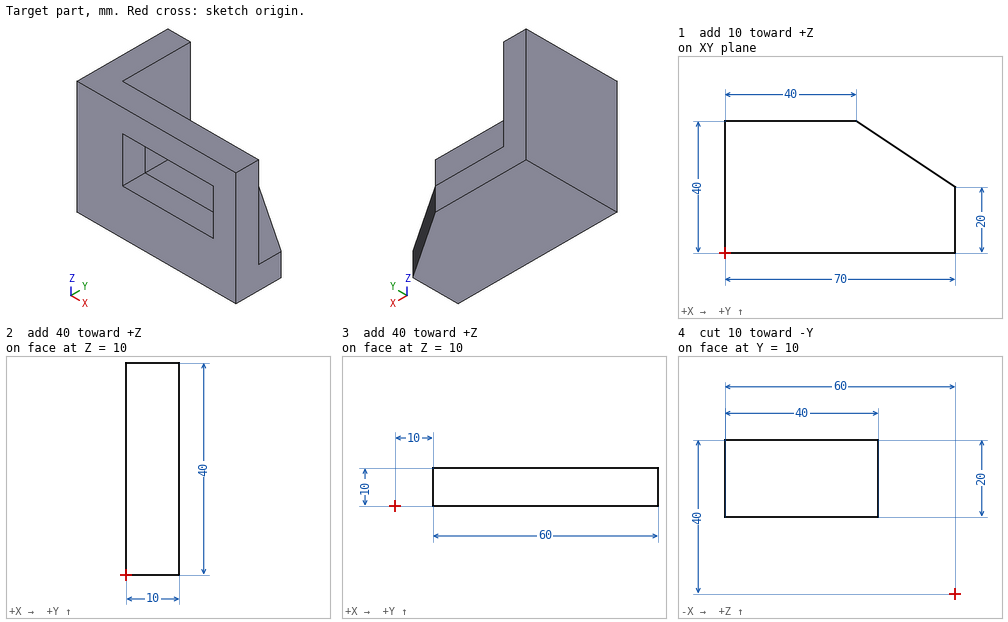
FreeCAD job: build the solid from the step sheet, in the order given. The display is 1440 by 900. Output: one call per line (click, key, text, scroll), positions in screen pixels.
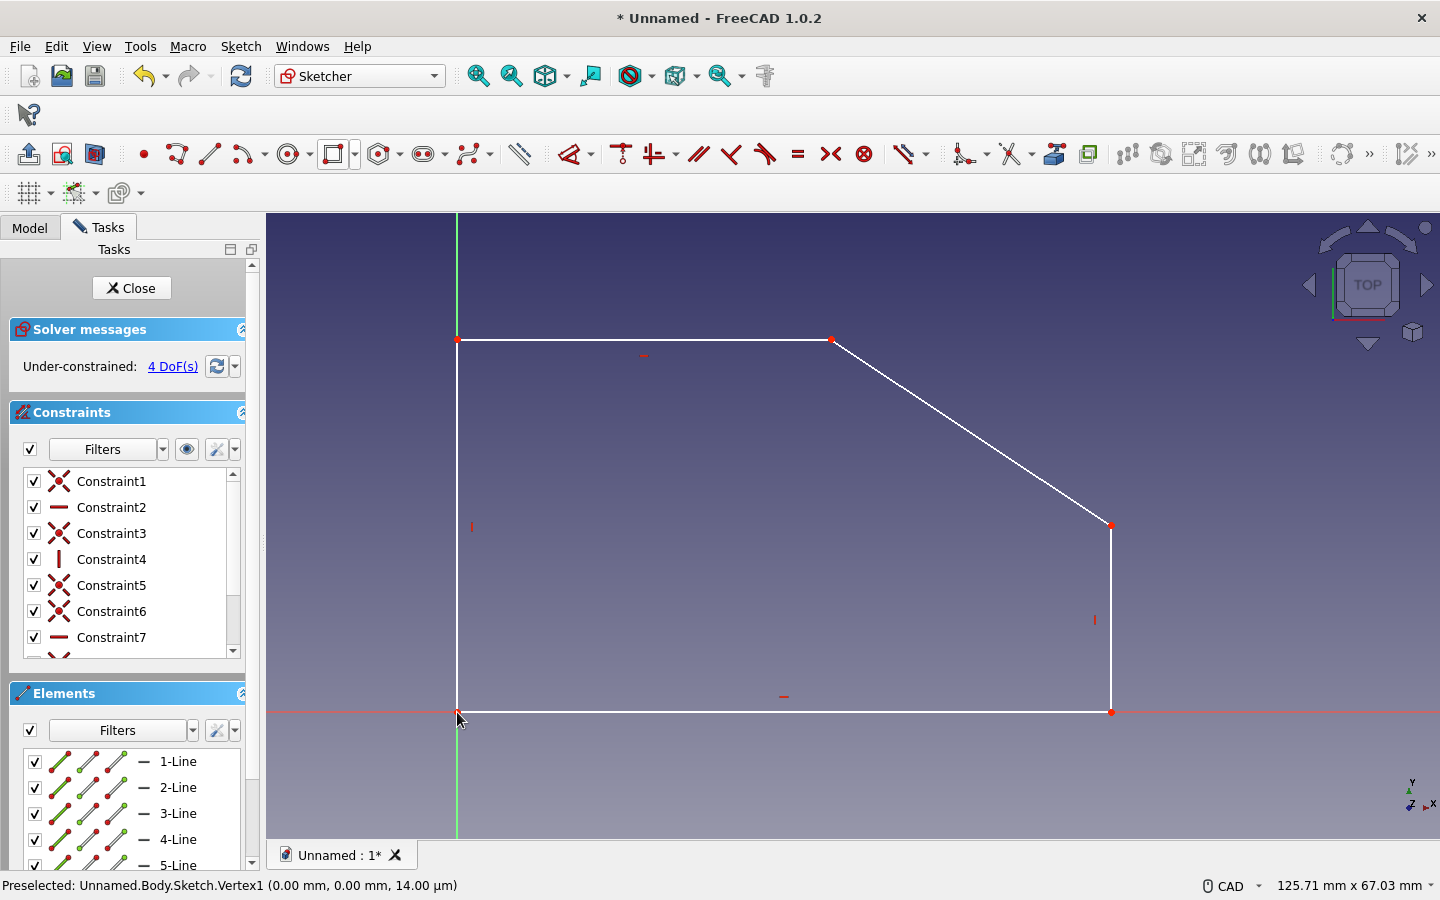
click(568, 154)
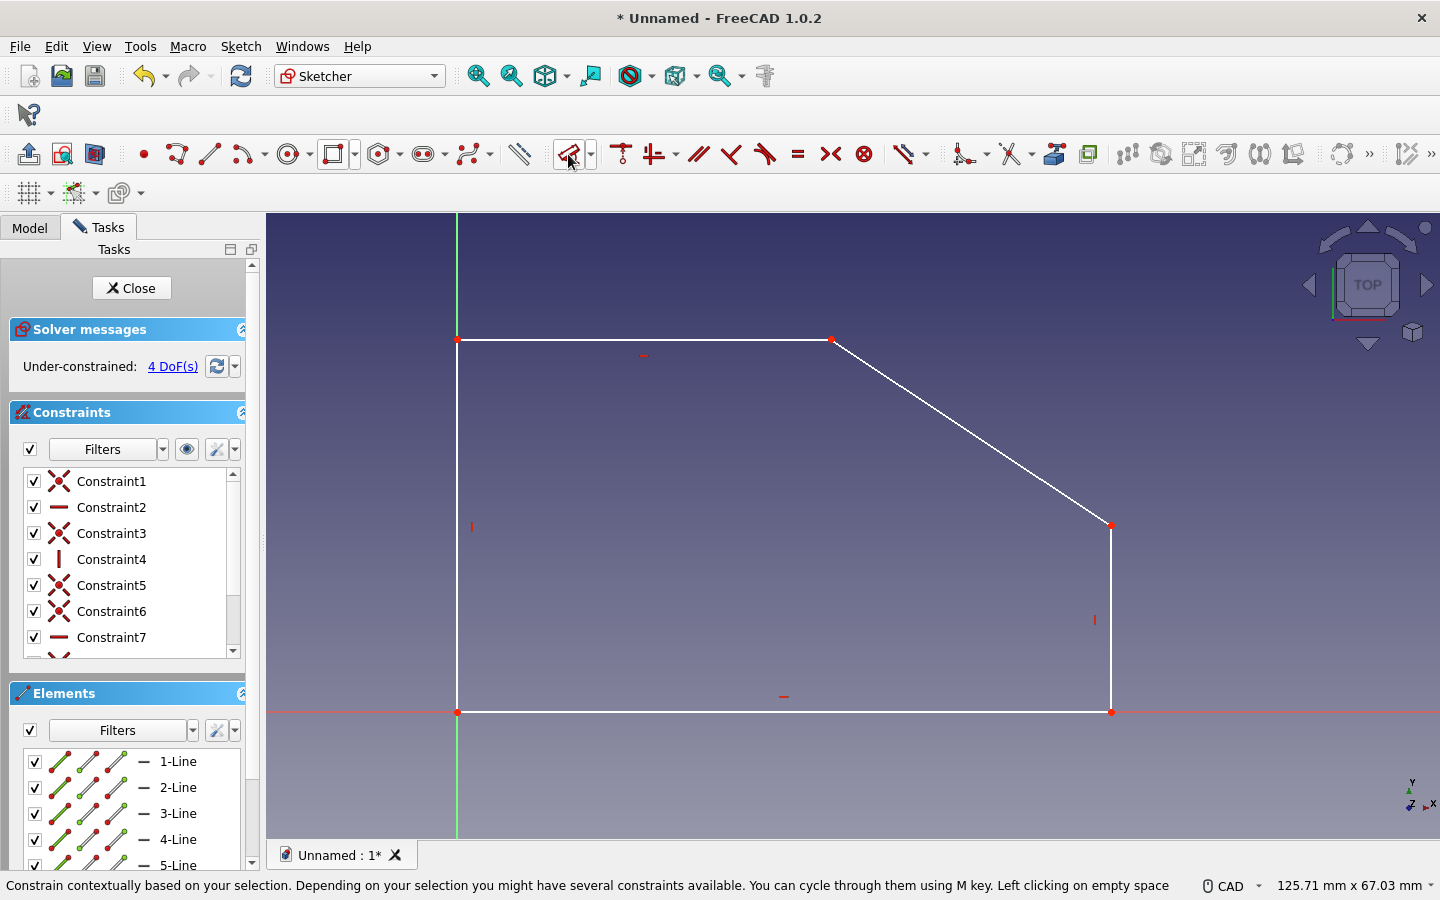
click(653, 712)
click(784, 746)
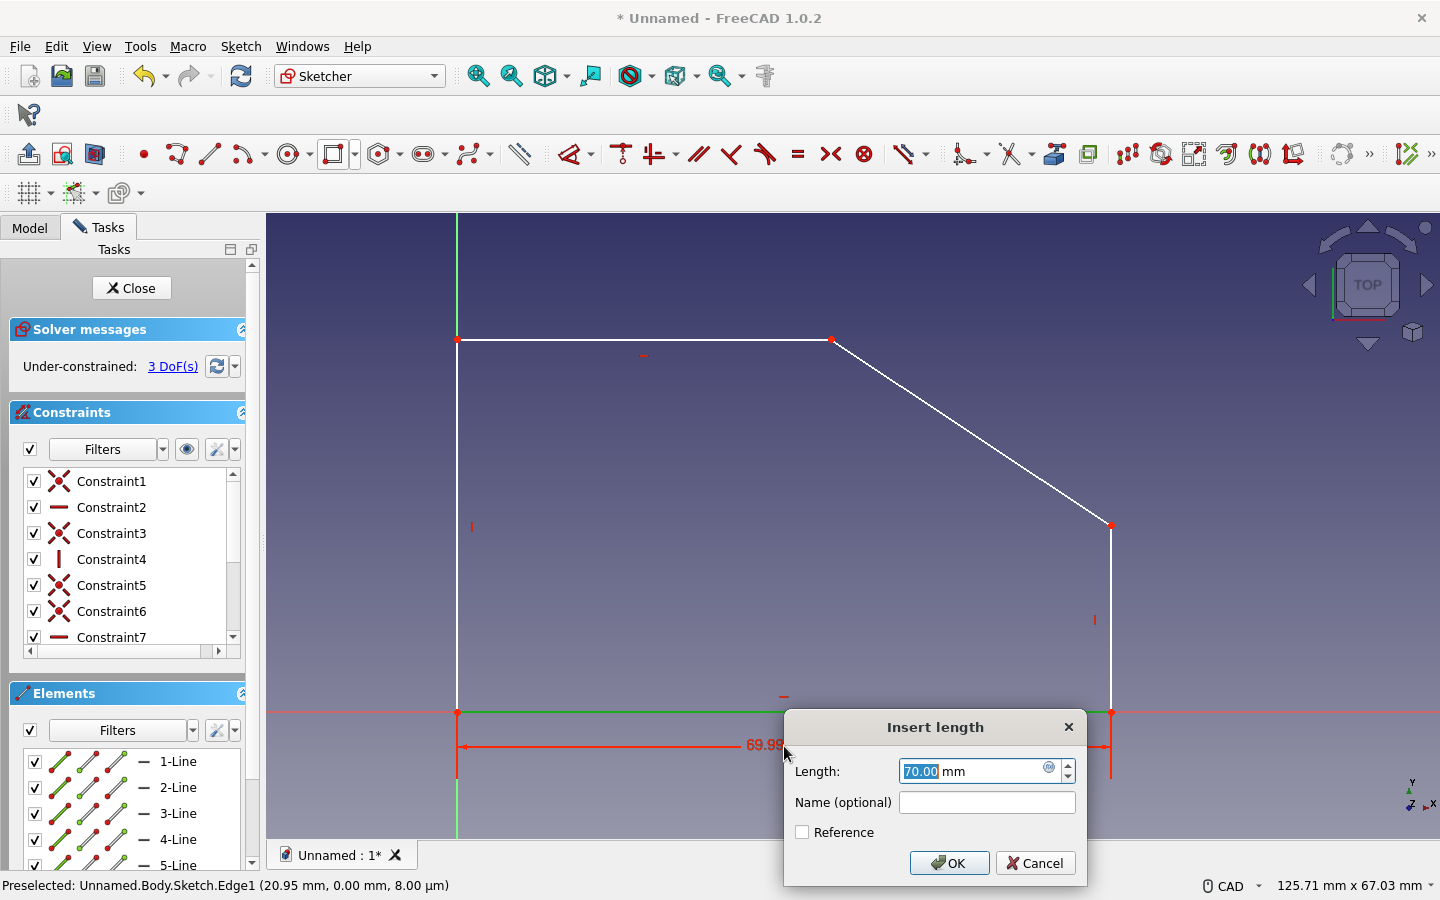
text(70)
key(Return)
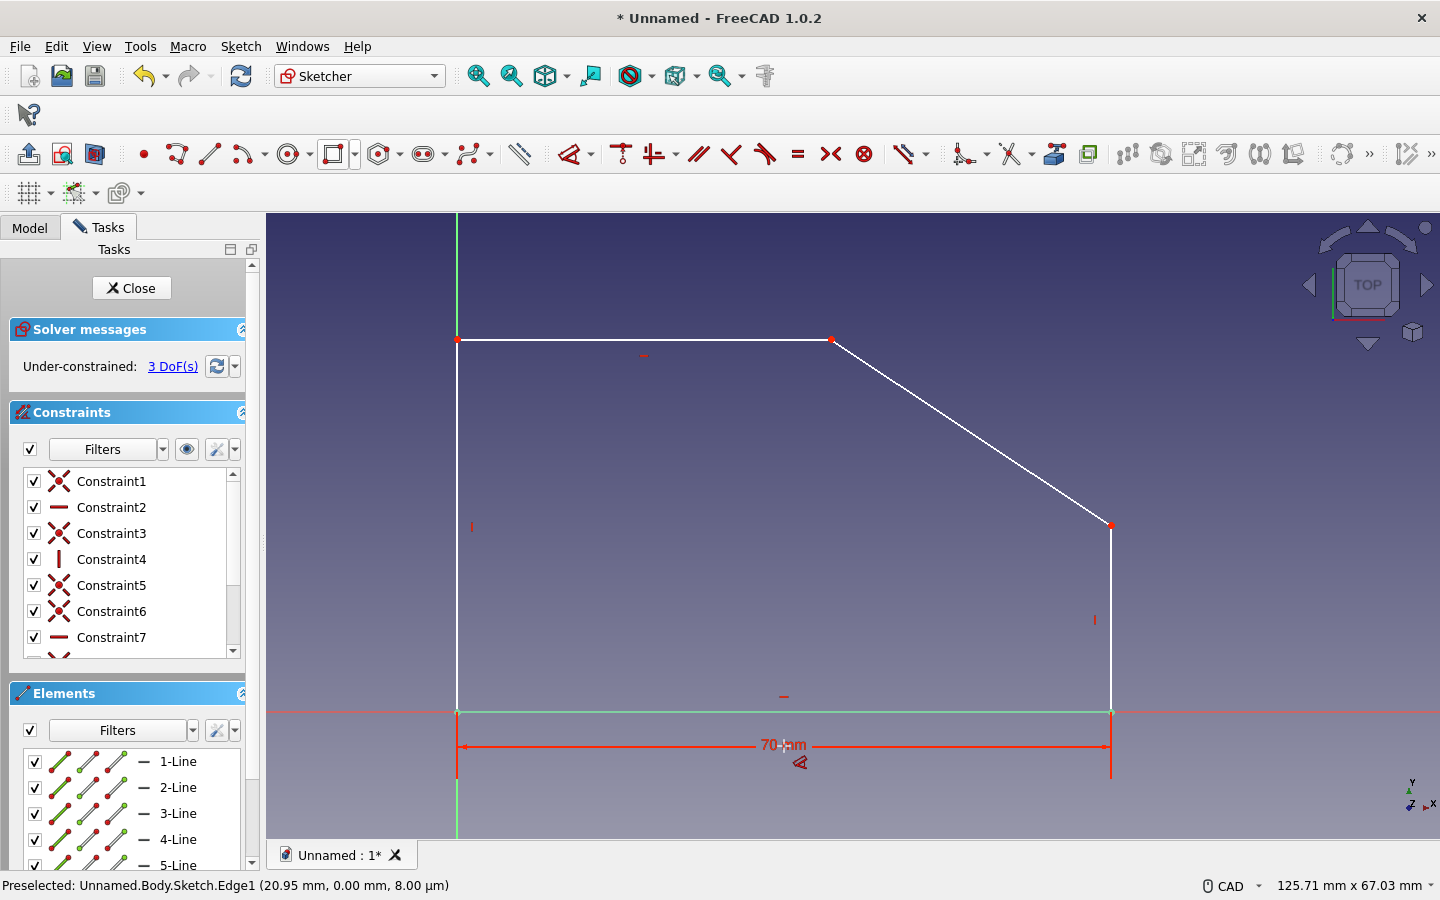
click(1111, 656)
click(1145, 619)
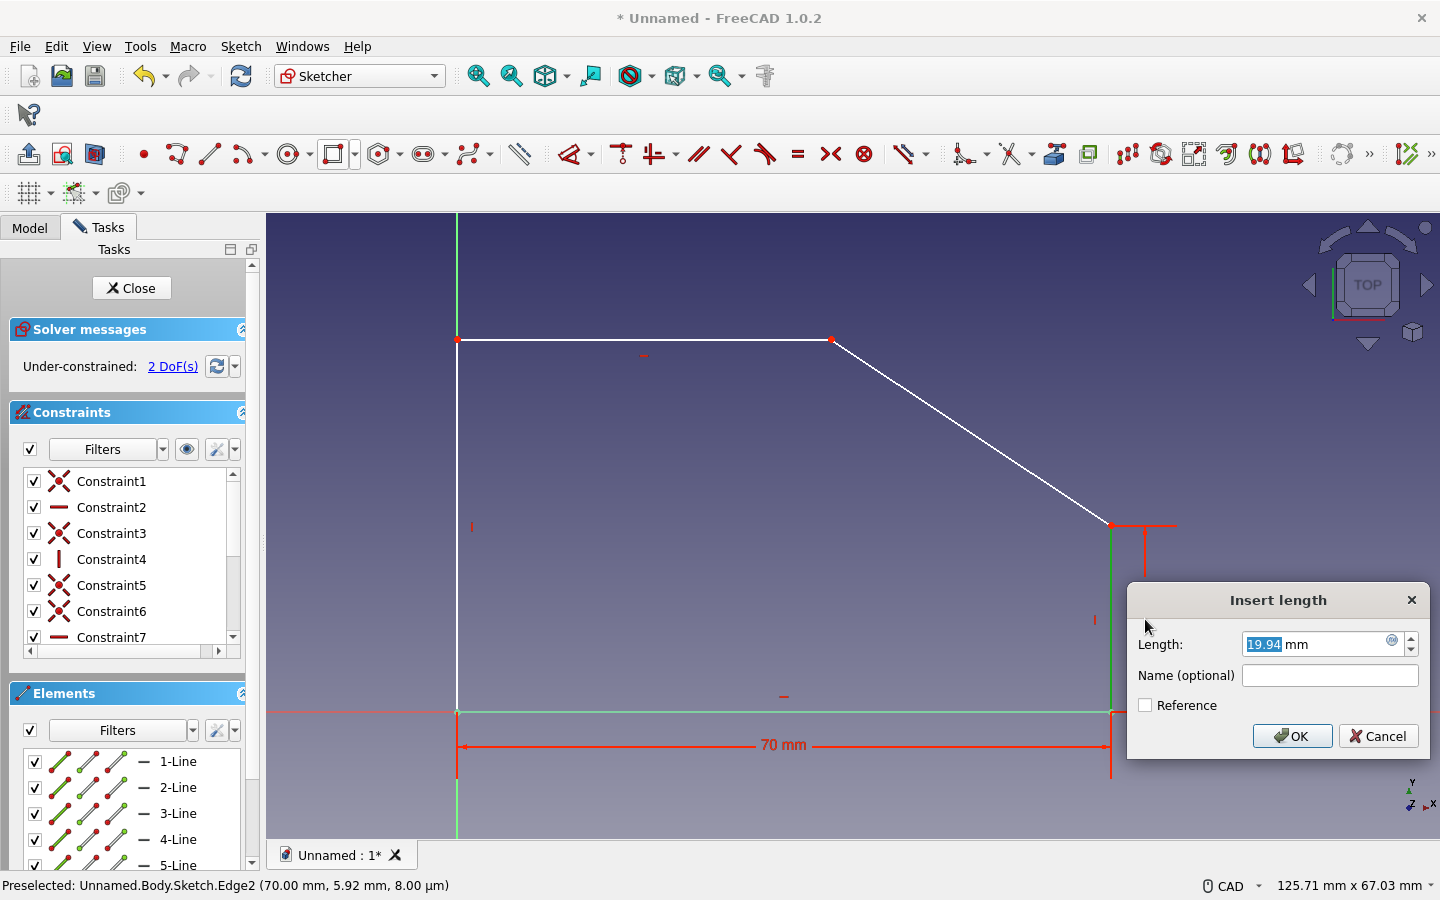
text(20)
key(Return)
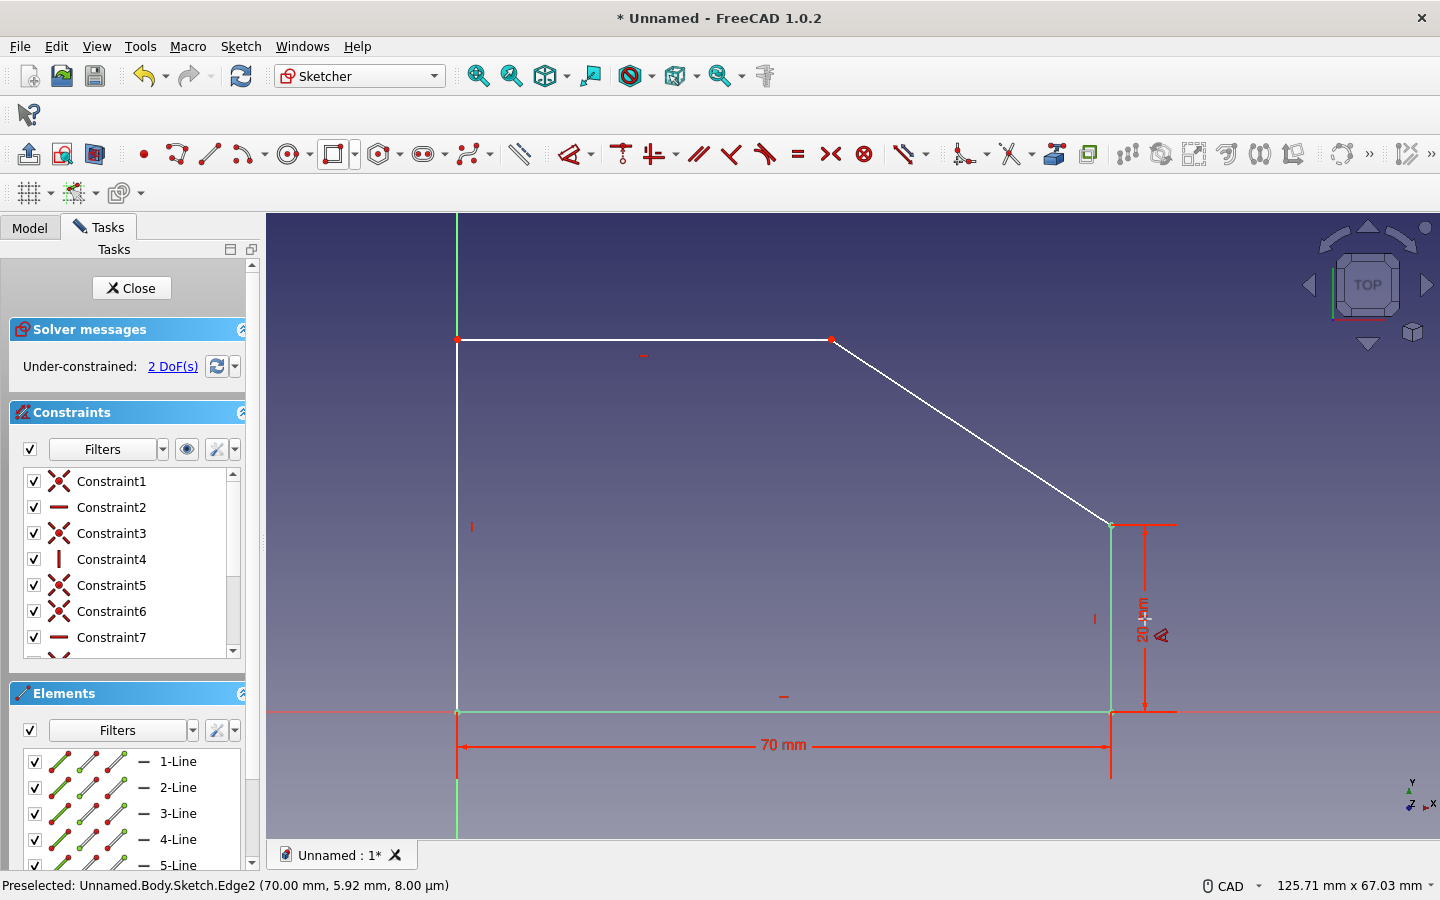
click(719, 340)
click(644, 306)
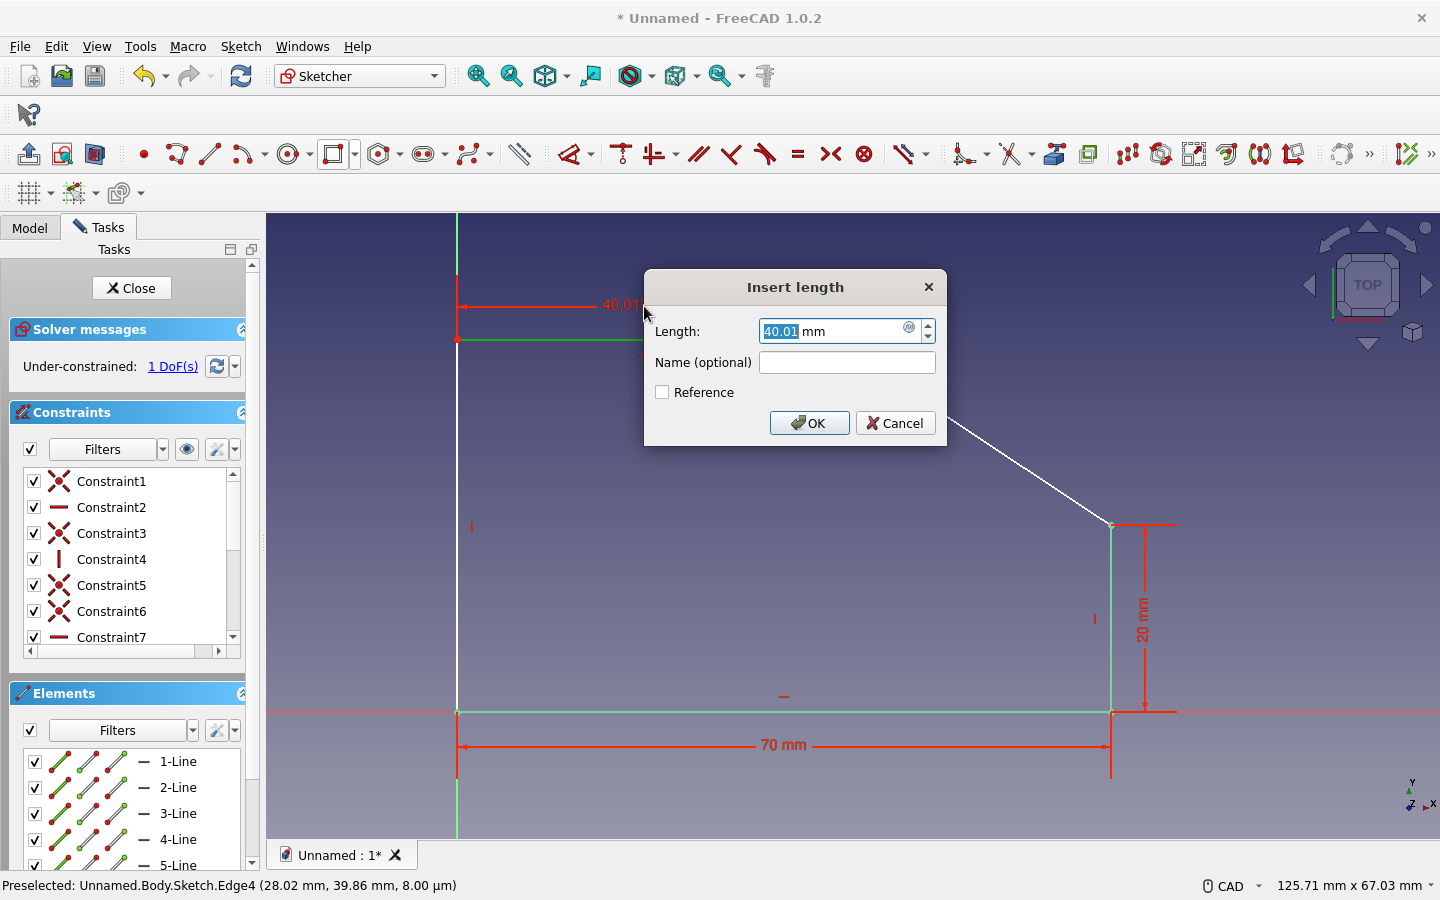
text(40)
key(Return)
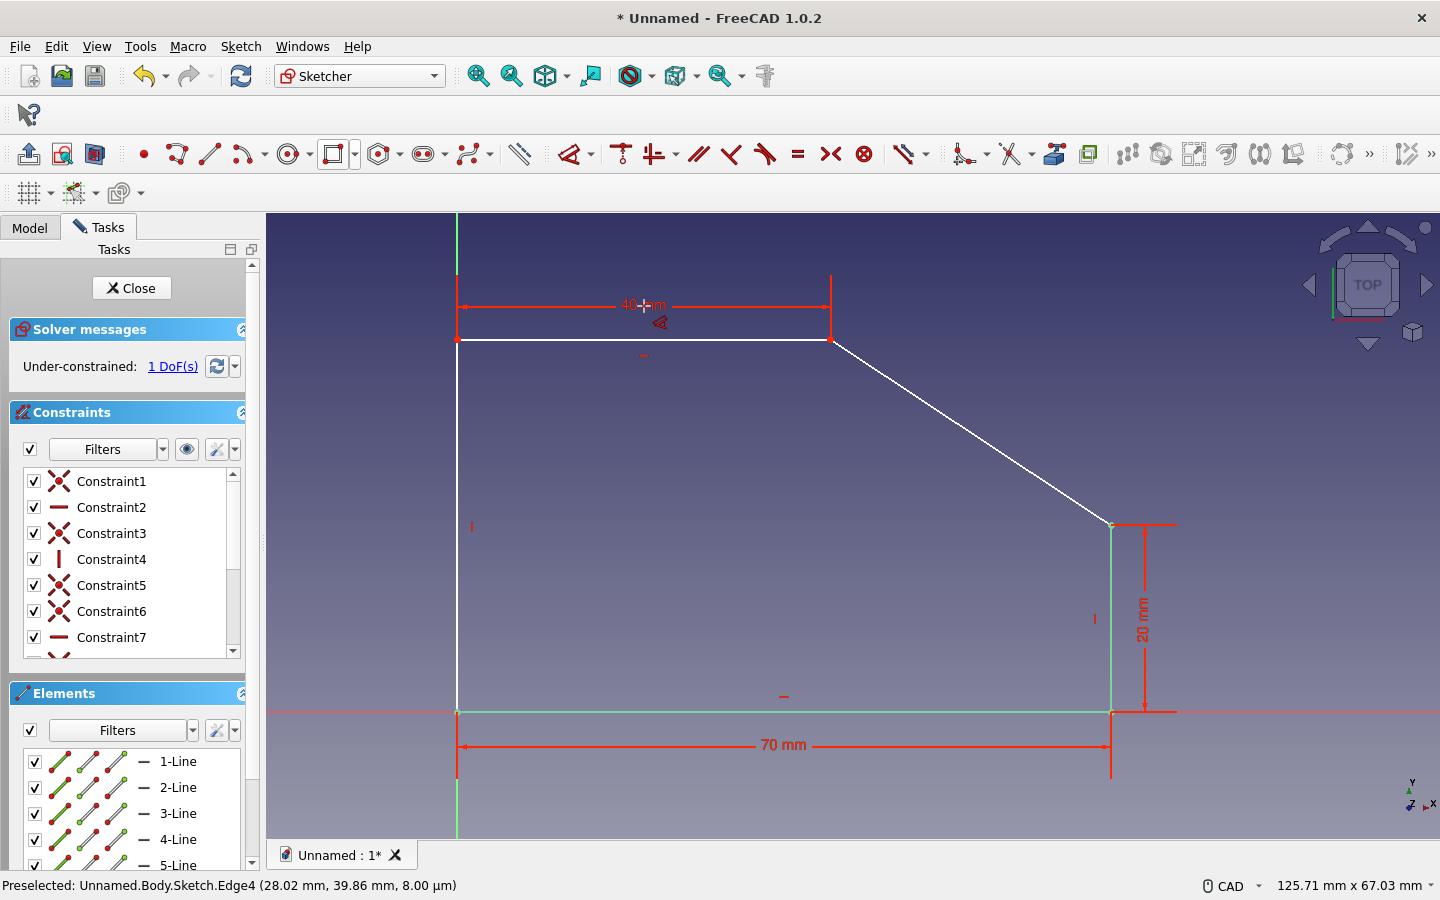
click(457, 452)
click(423, 526)